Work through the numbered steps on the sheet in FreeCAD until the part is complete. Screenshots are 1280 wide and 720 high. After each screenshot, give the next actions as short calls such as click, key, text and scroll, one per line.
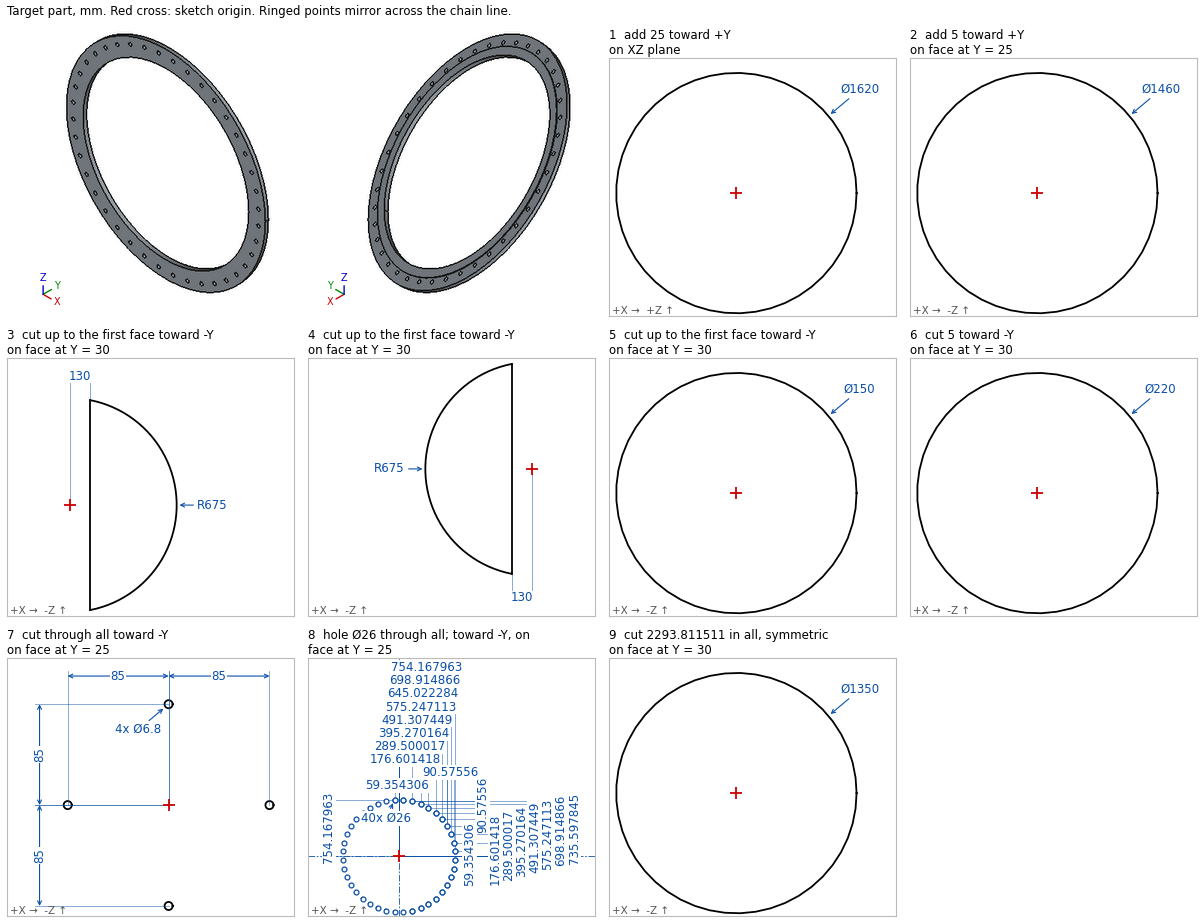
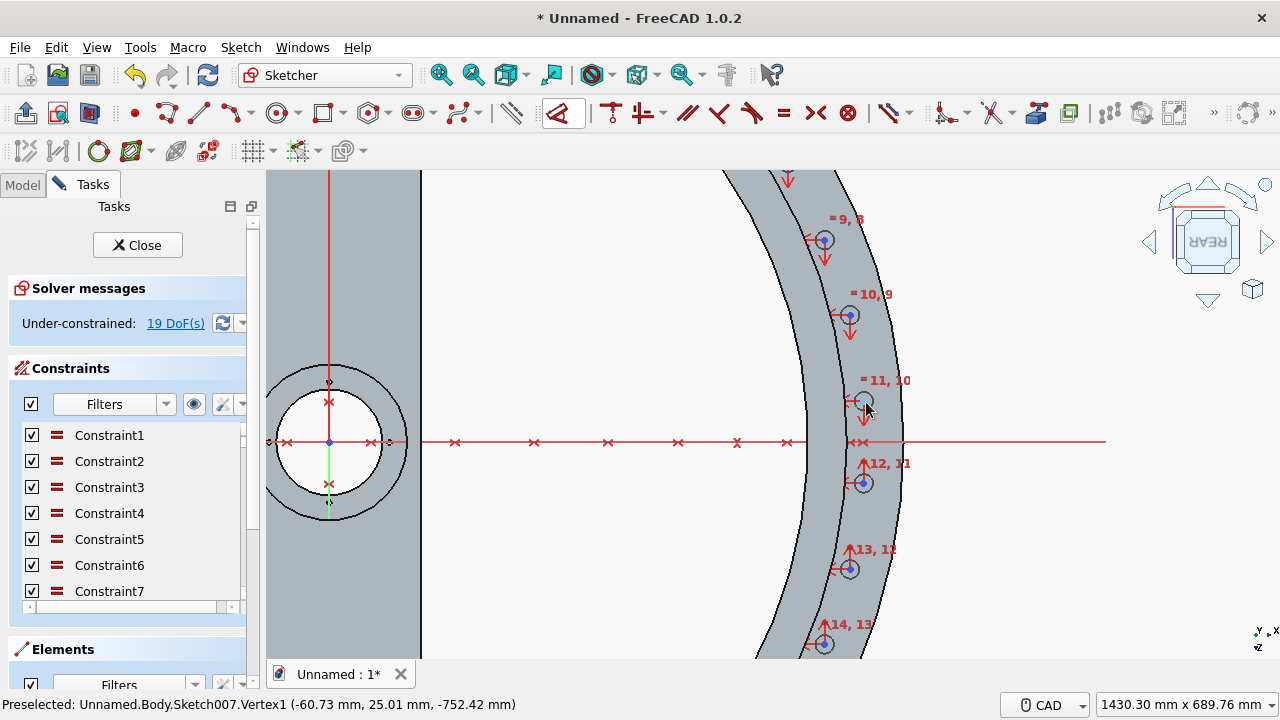
click(864, 401)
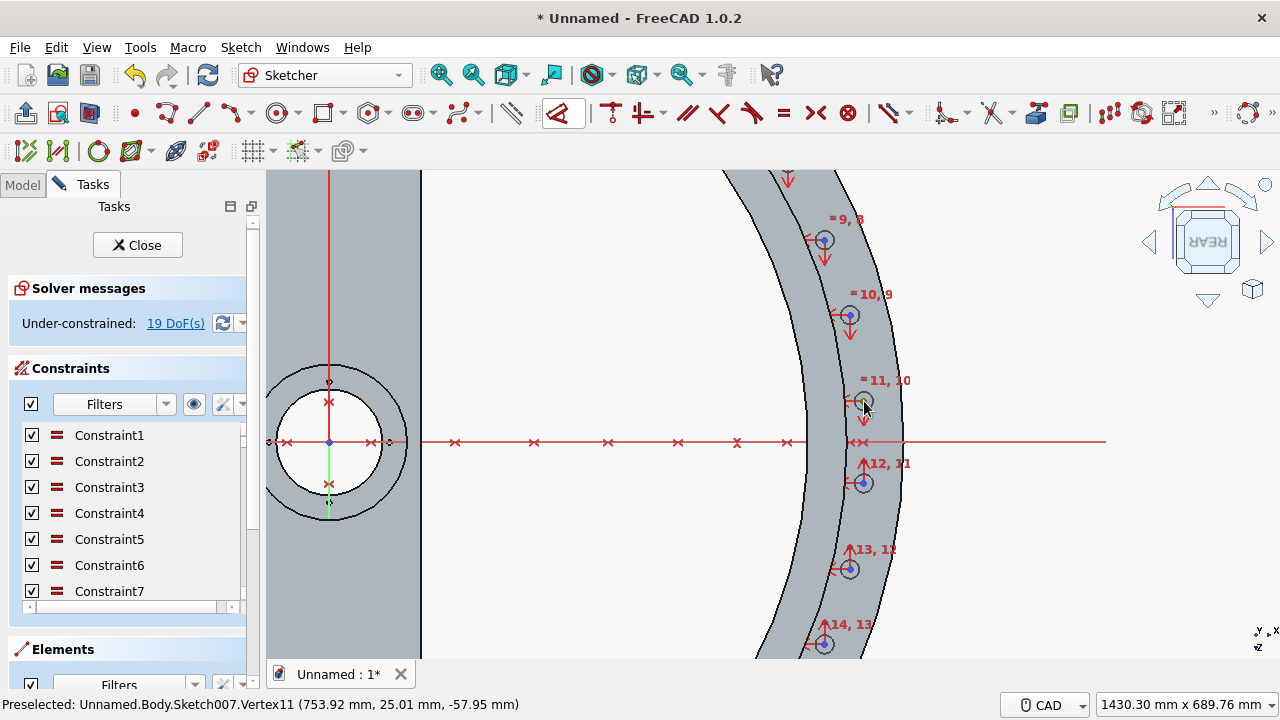
key(i)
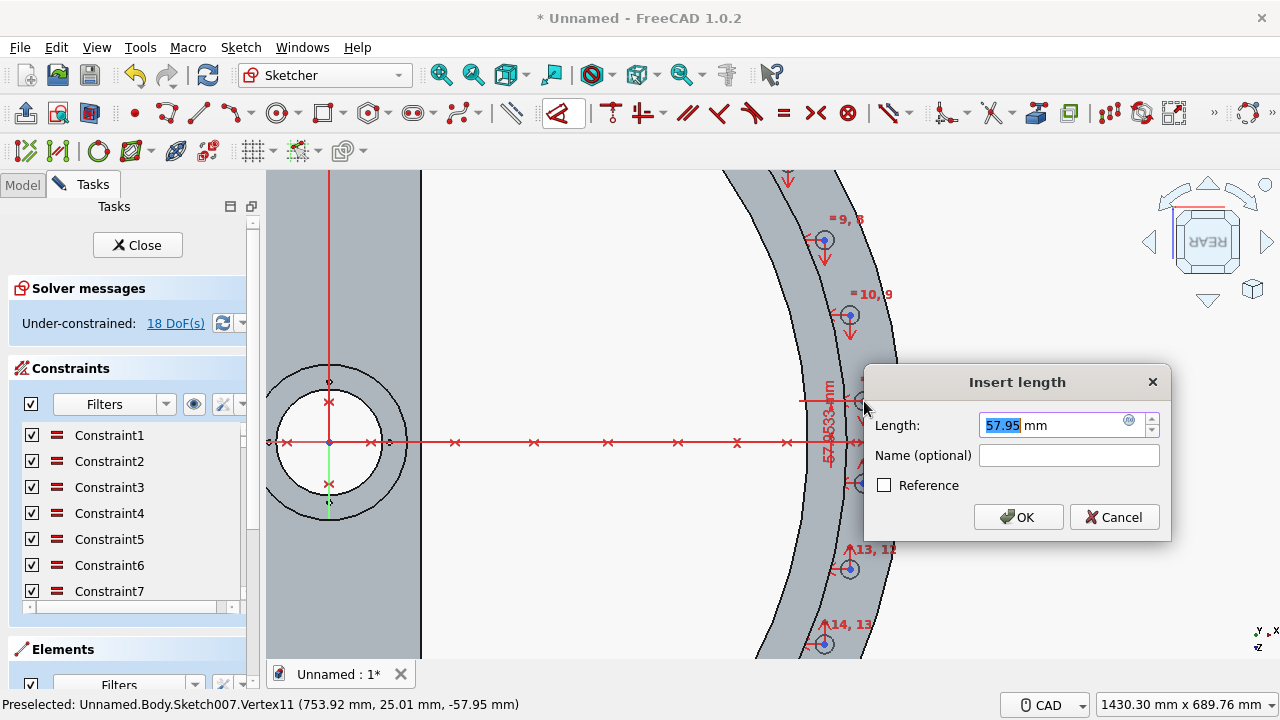
text(59.354306)
key(Return)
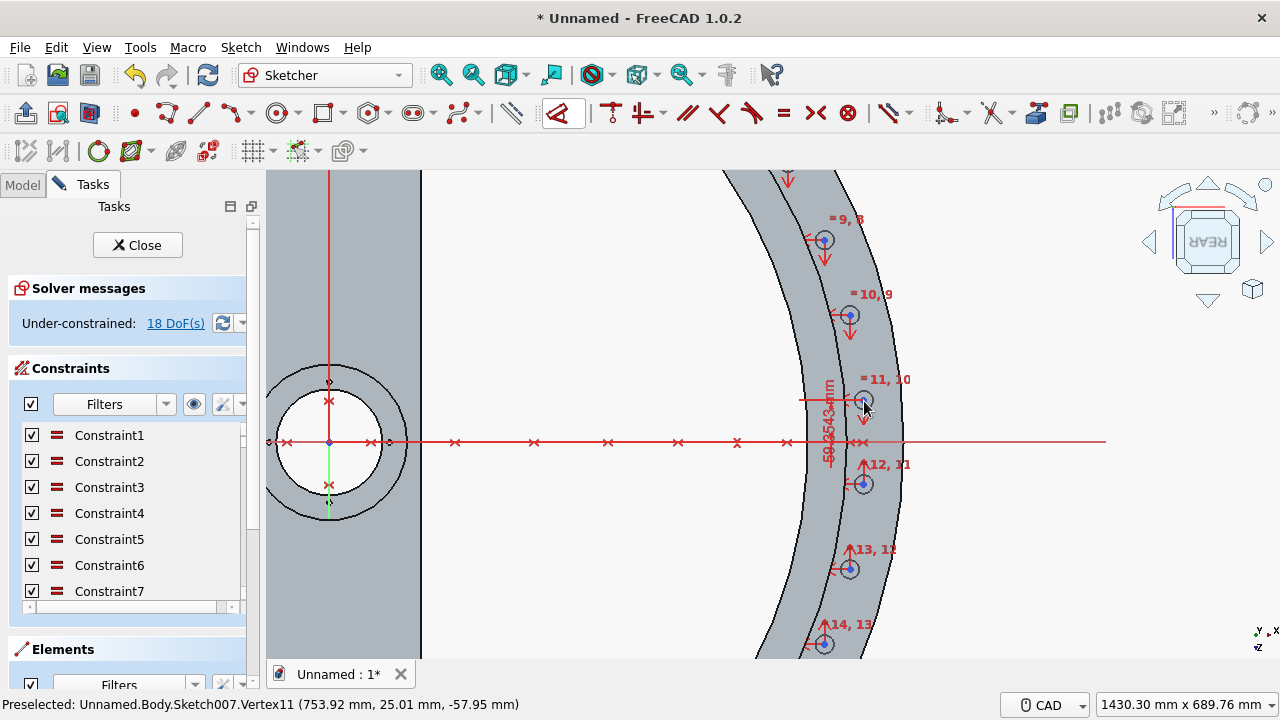
scroll(866, 403, down, 6)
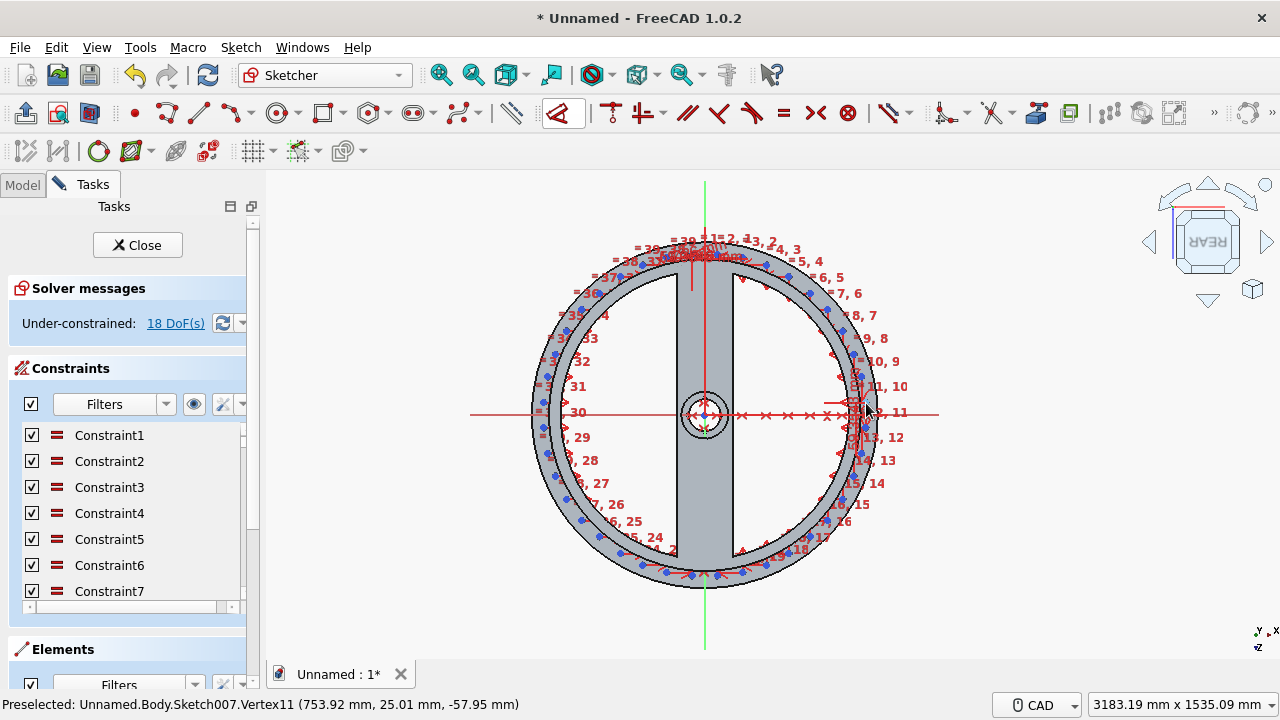
scroll(743, 258, up, 4)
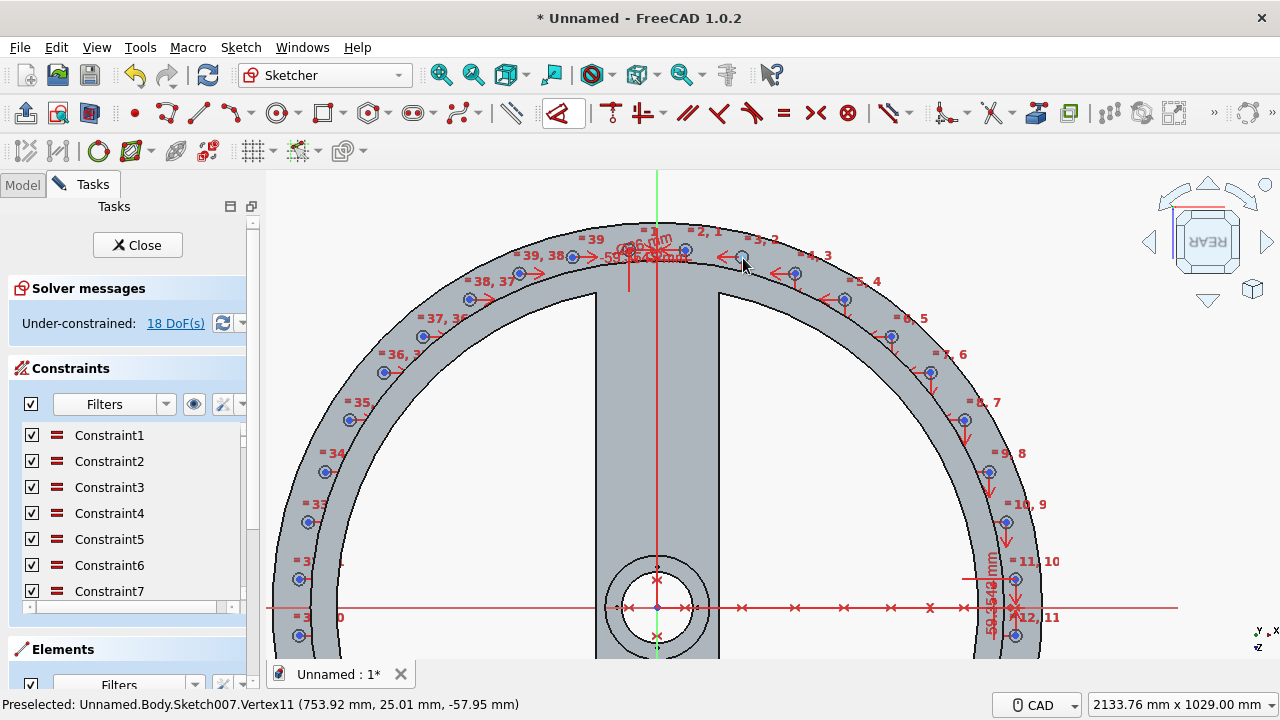
click(742, 257)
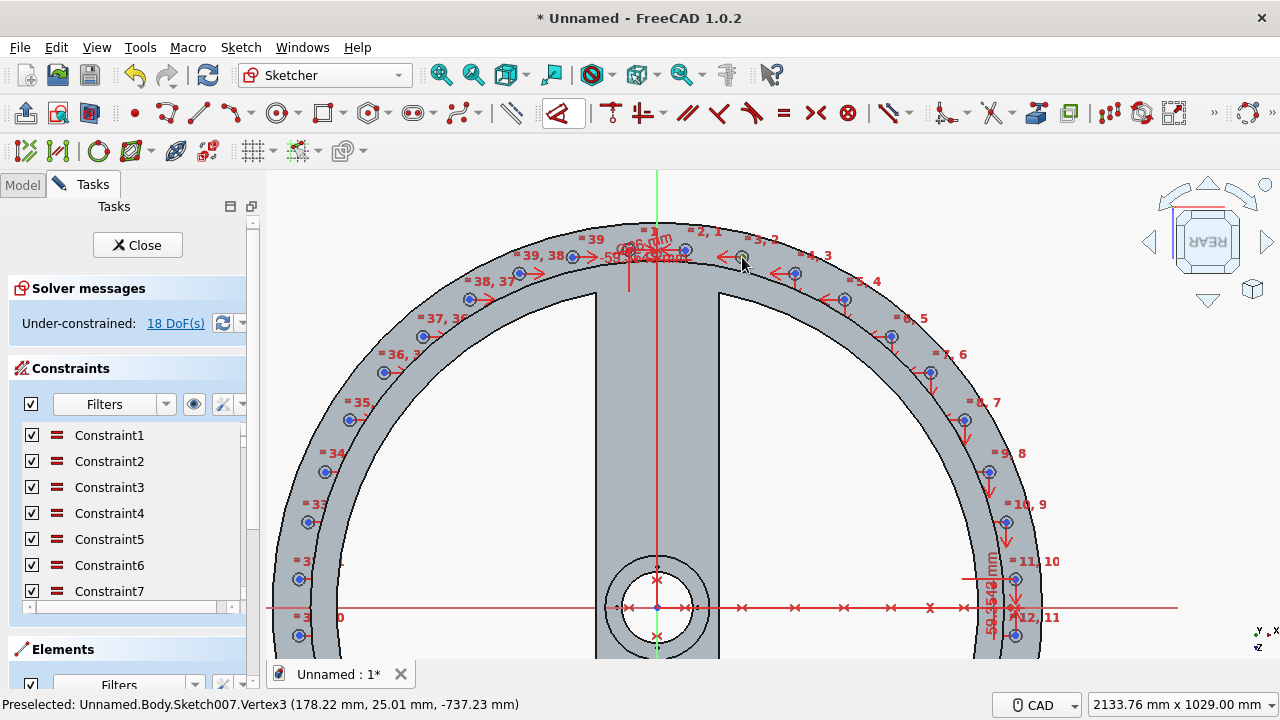
click(845, 300)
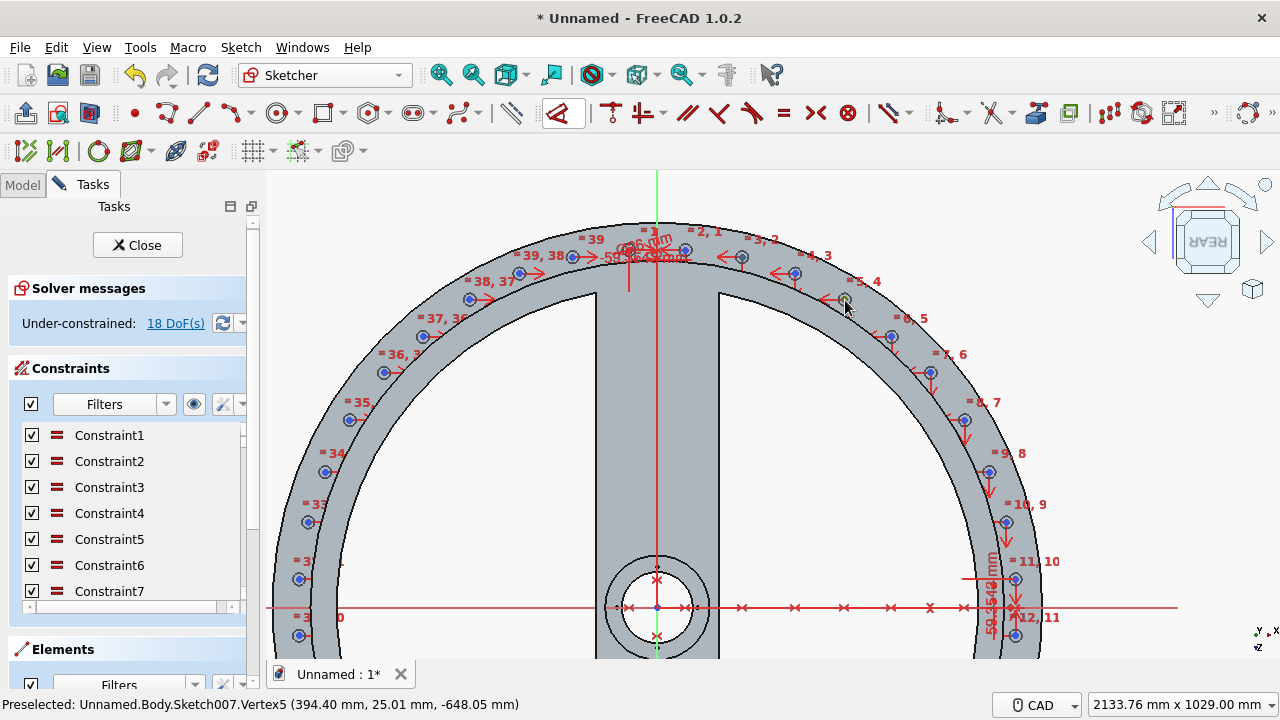
click(580, 114)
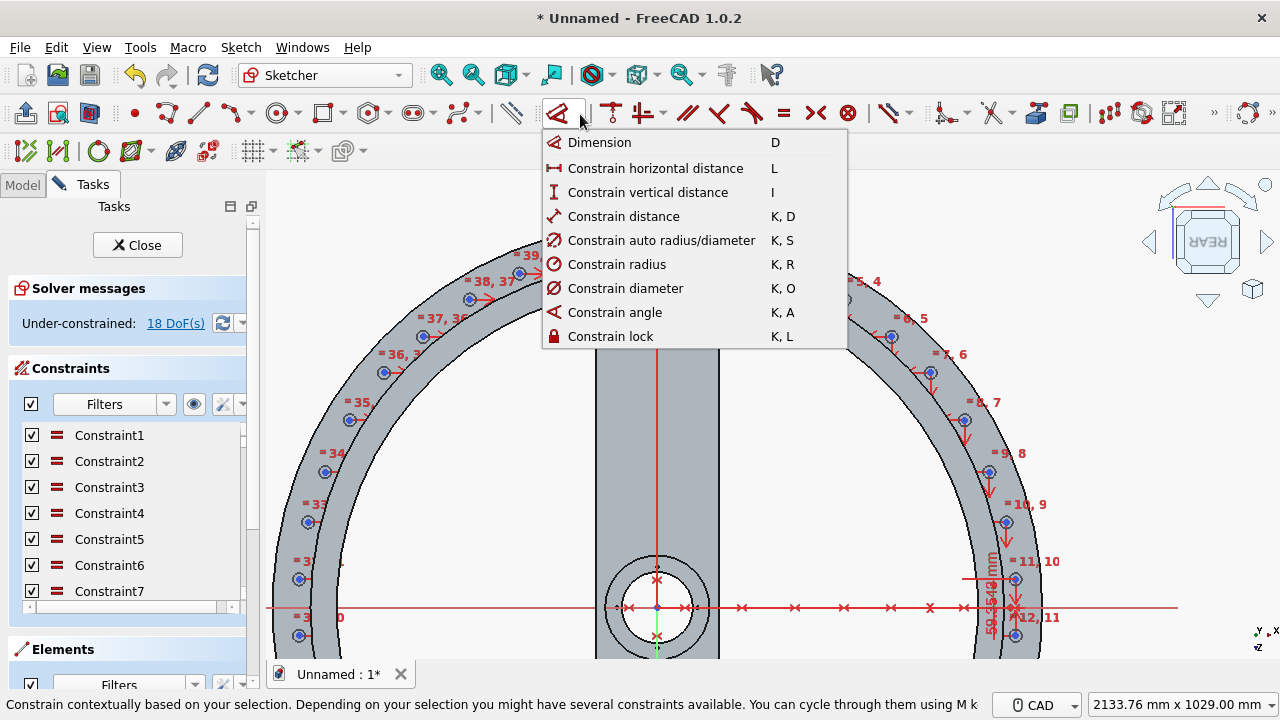
click(695, 192)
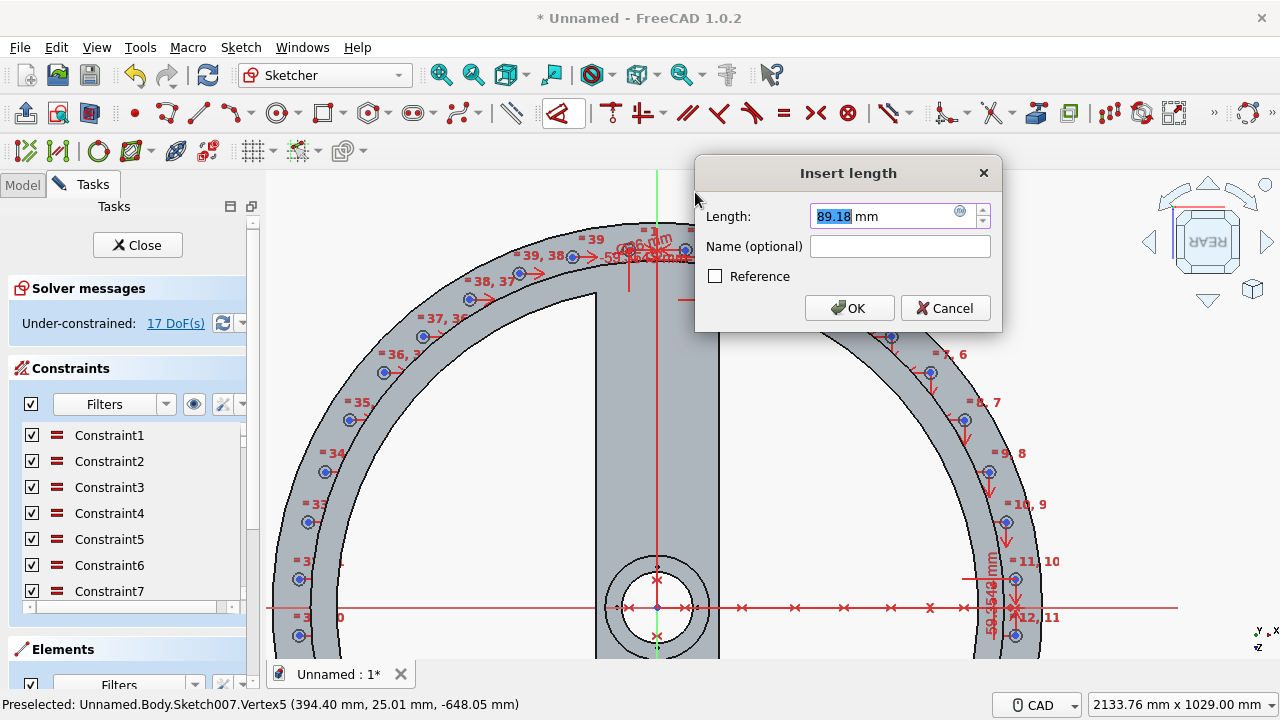
text(90.57556)
key(Return)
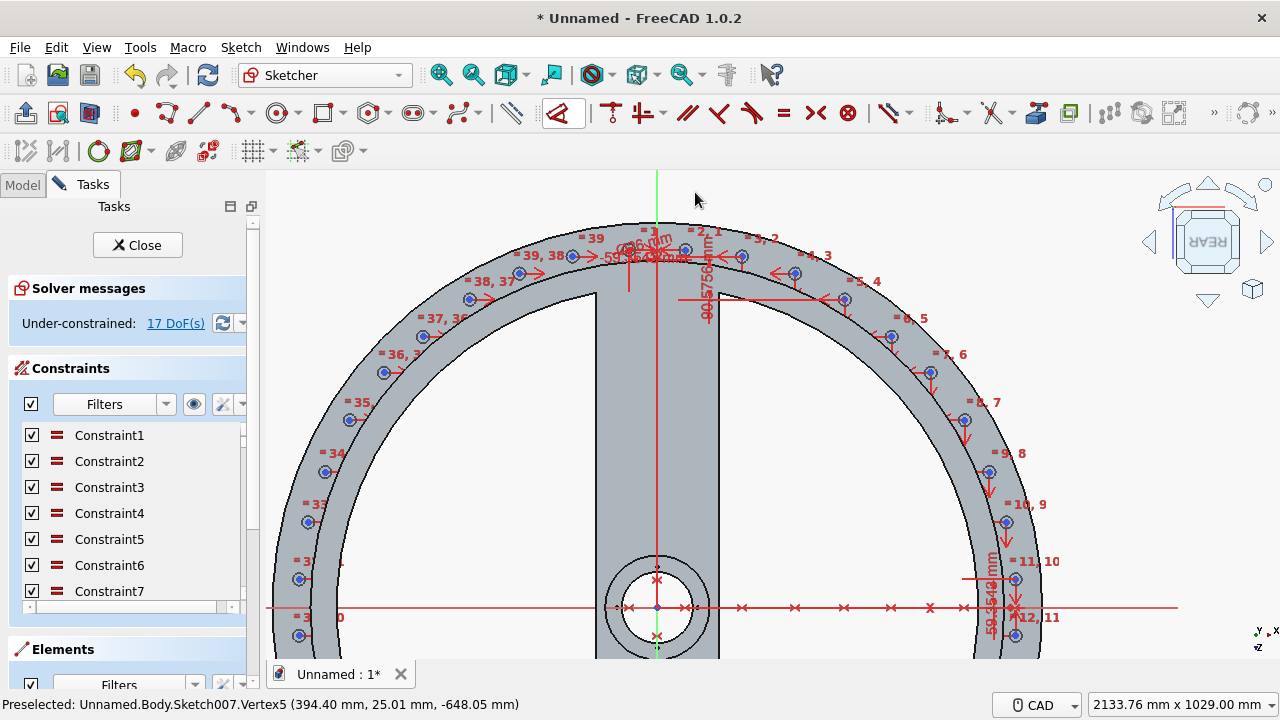
click(965, 420)